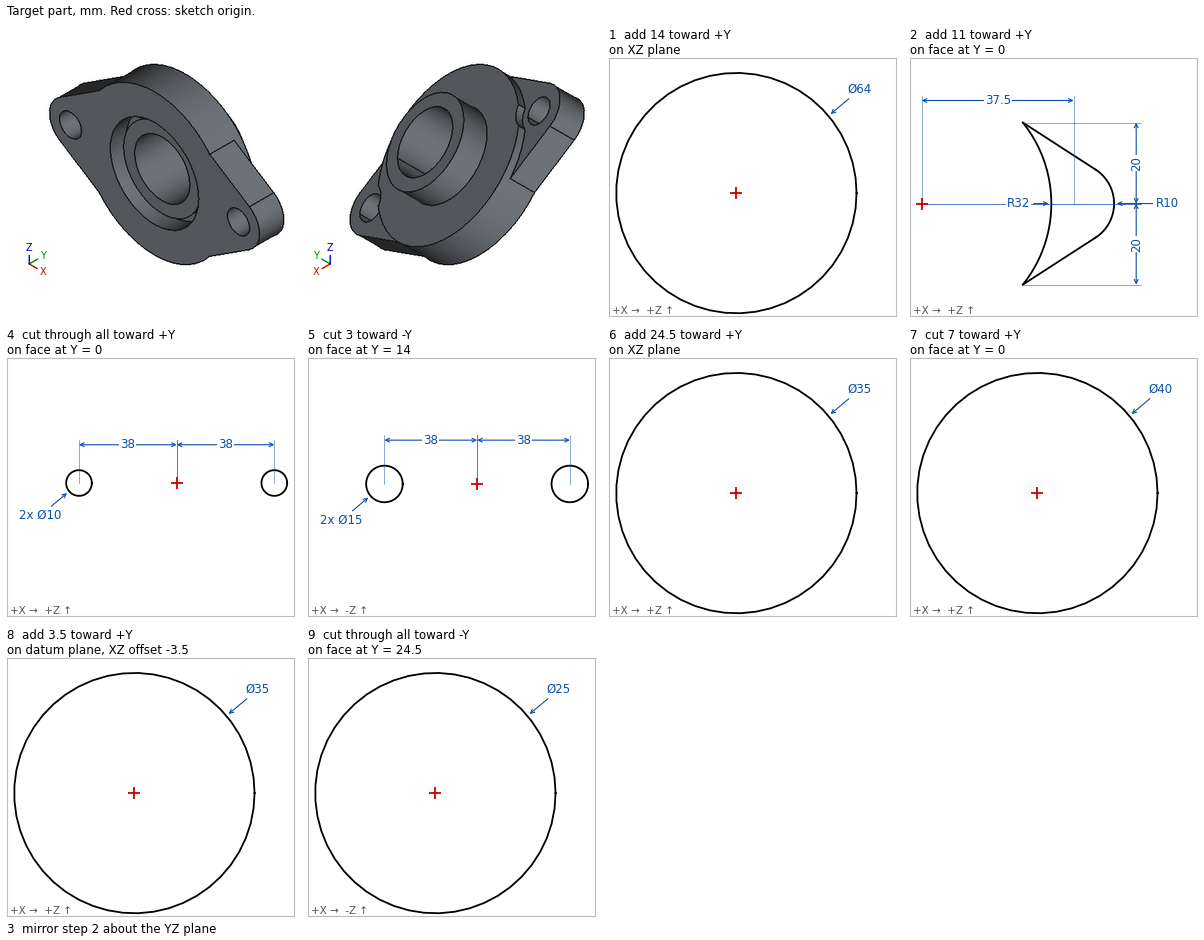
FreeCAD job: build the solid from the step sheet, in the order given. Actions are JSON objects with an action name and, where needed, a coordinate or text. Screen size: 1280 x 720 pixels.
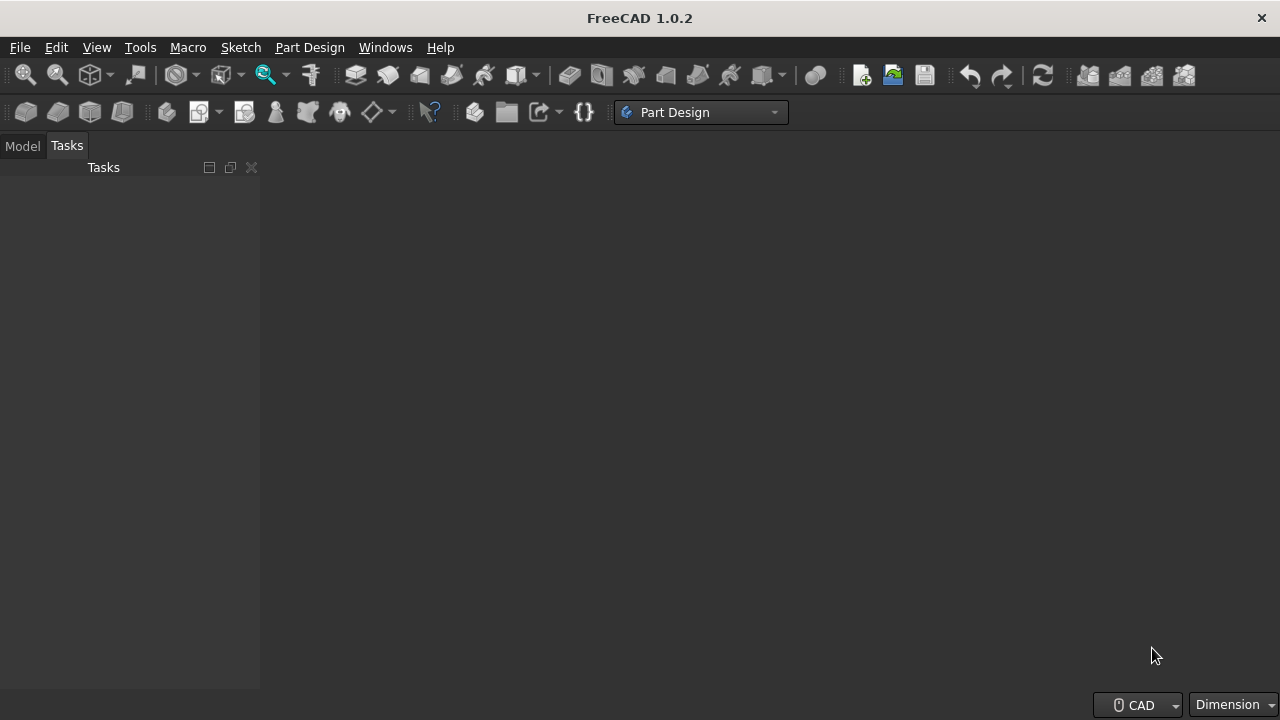
{"action": "left_click", "coordinate": [862, 76]}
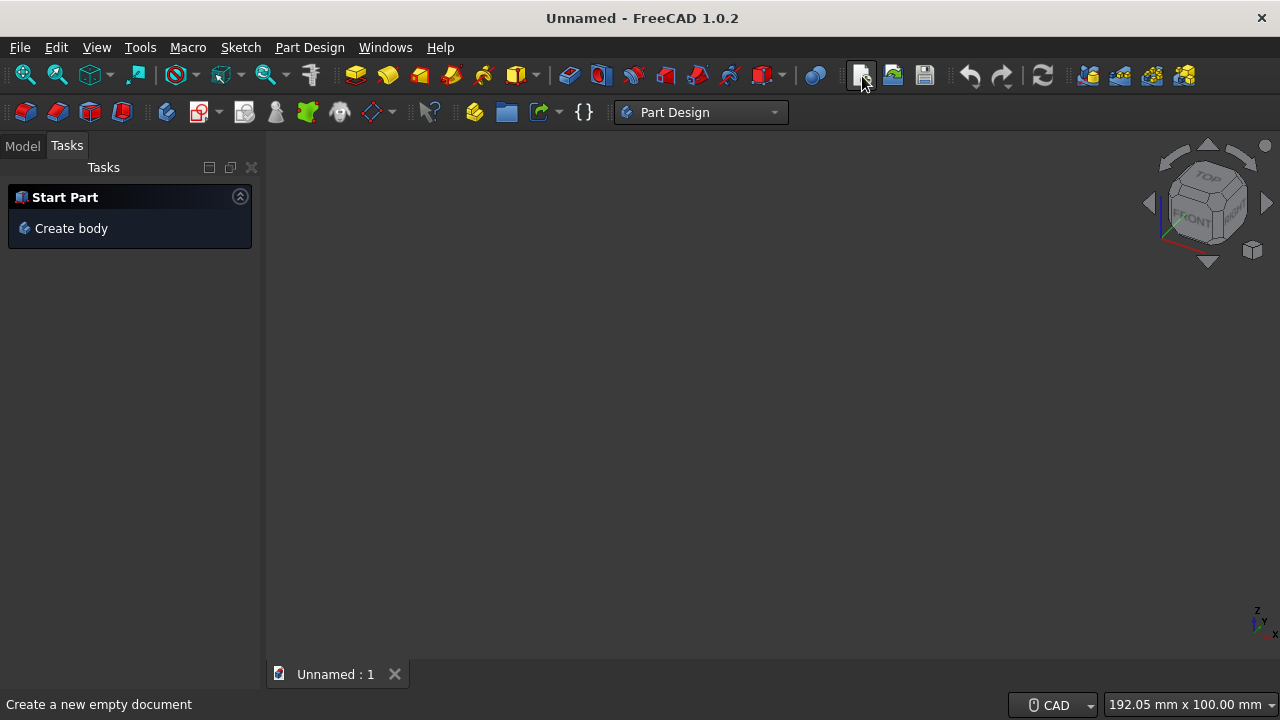
{"action": "left_click", "coordinate": [200, 112]}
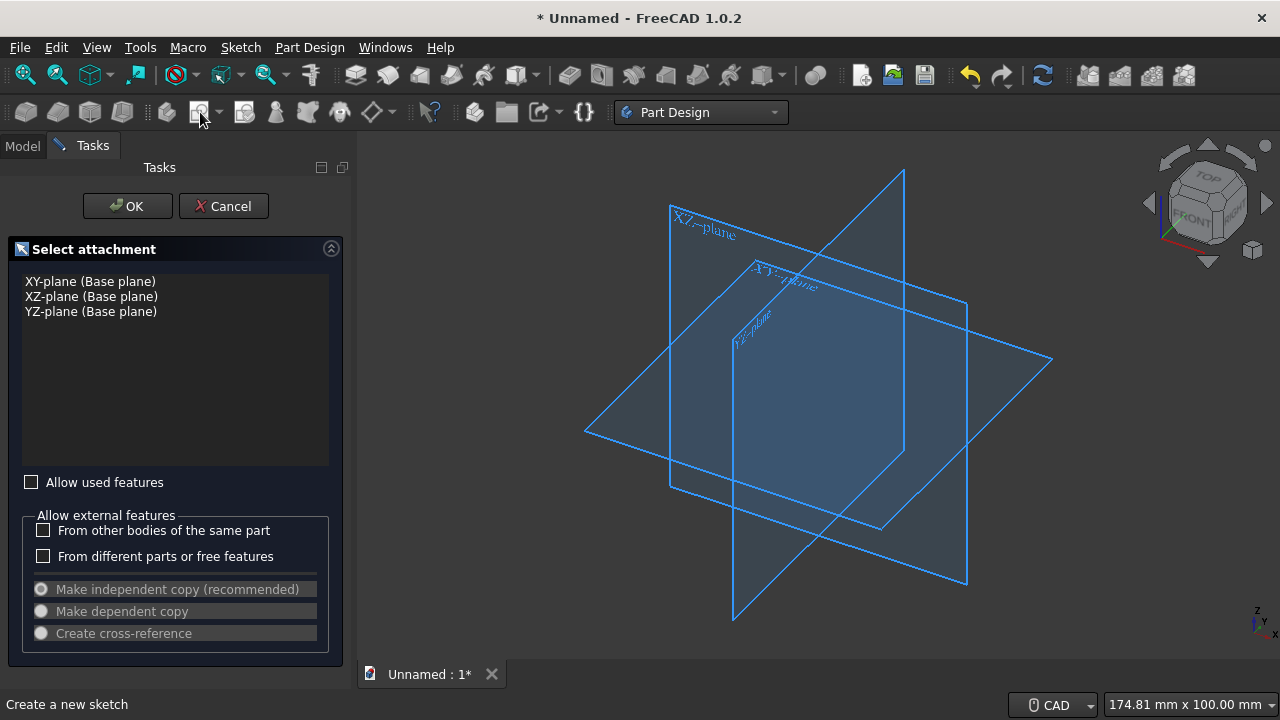
{"action": "left_click", "coordinate": [82, 296]}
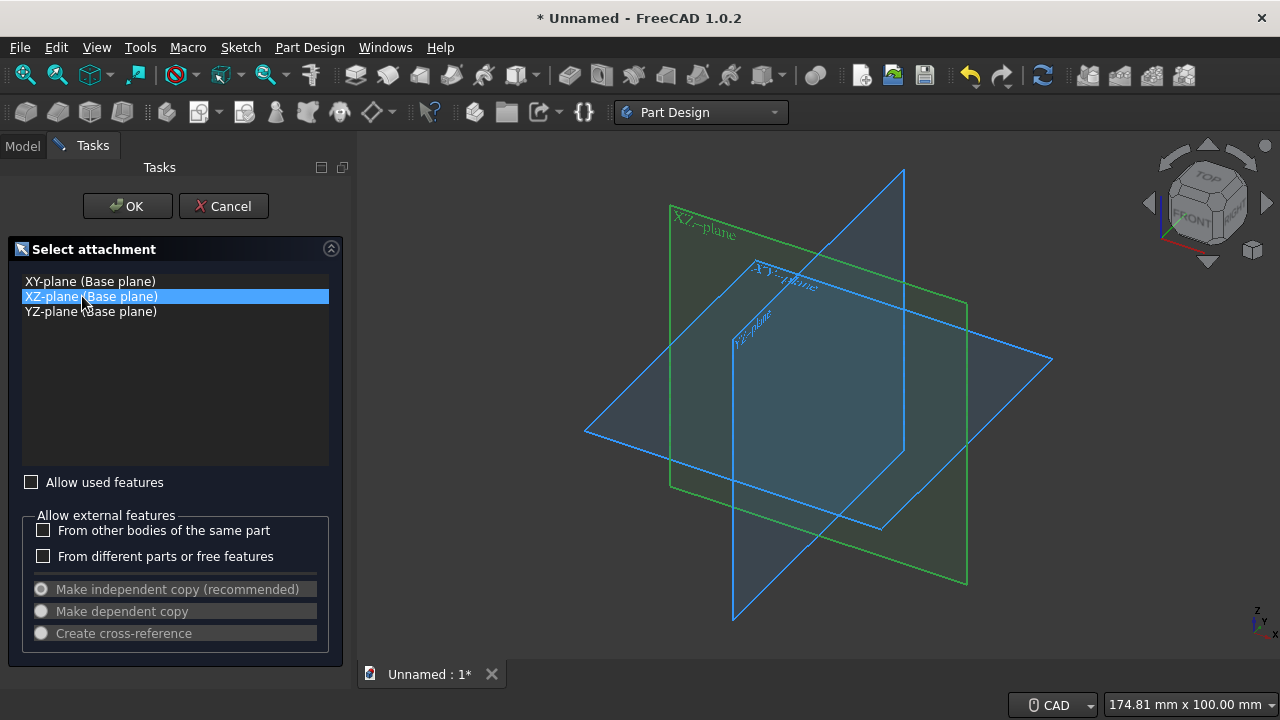
{"action": "left_click", "coordinate": [128, 206]}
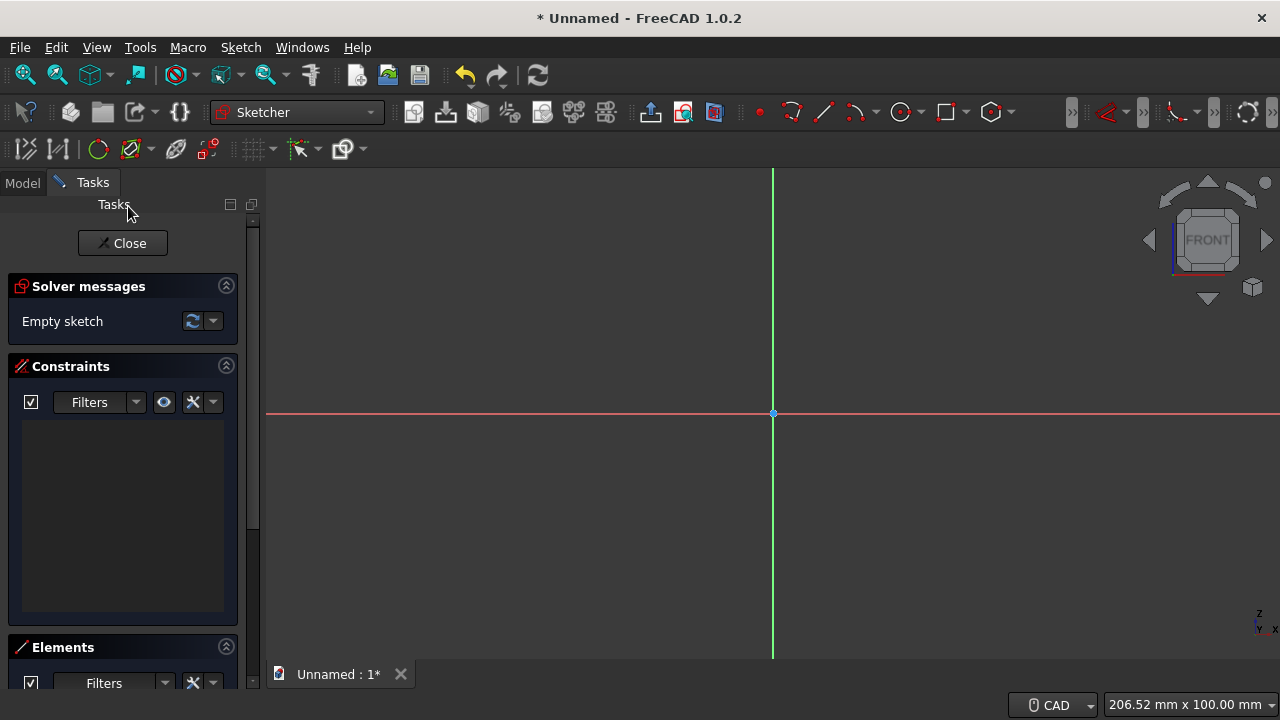
{"action": "key", "text": "g c"}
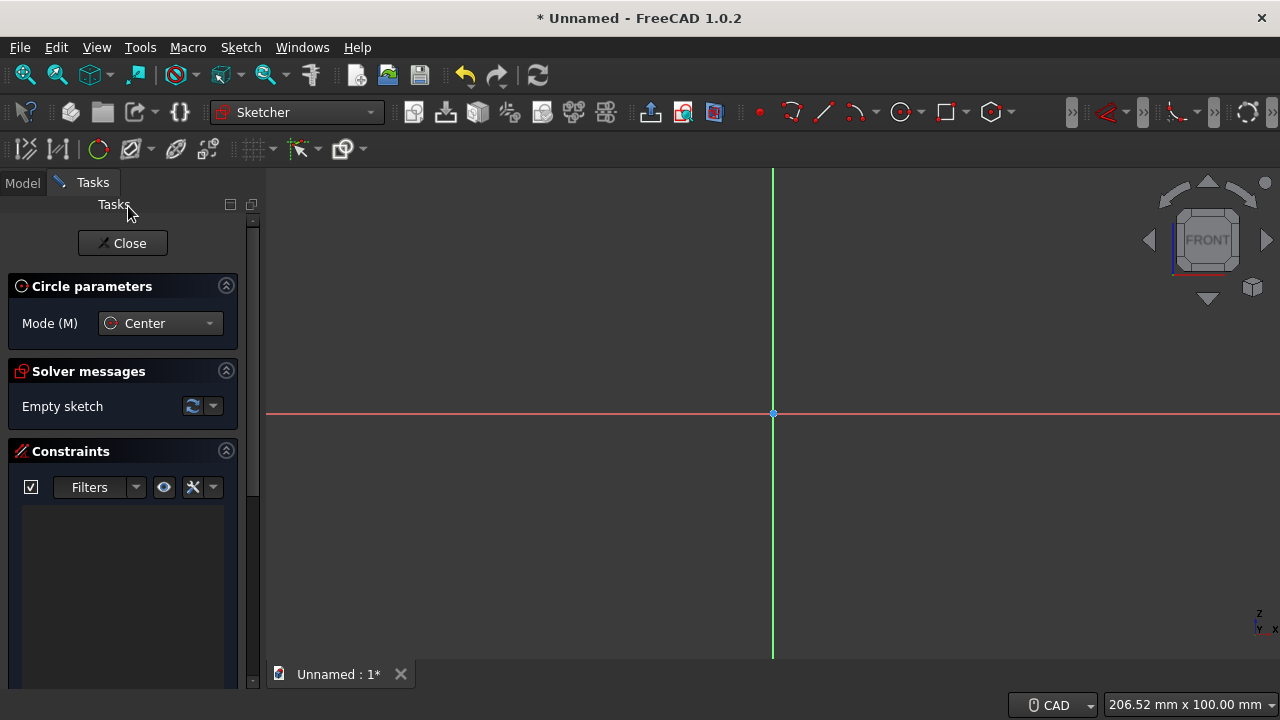
{"action": "left_click", "coordinate": [773, 414]}
{"action": "left_click", "coordinate": [884, 302]}
{"action": "key", "text": "Escape"}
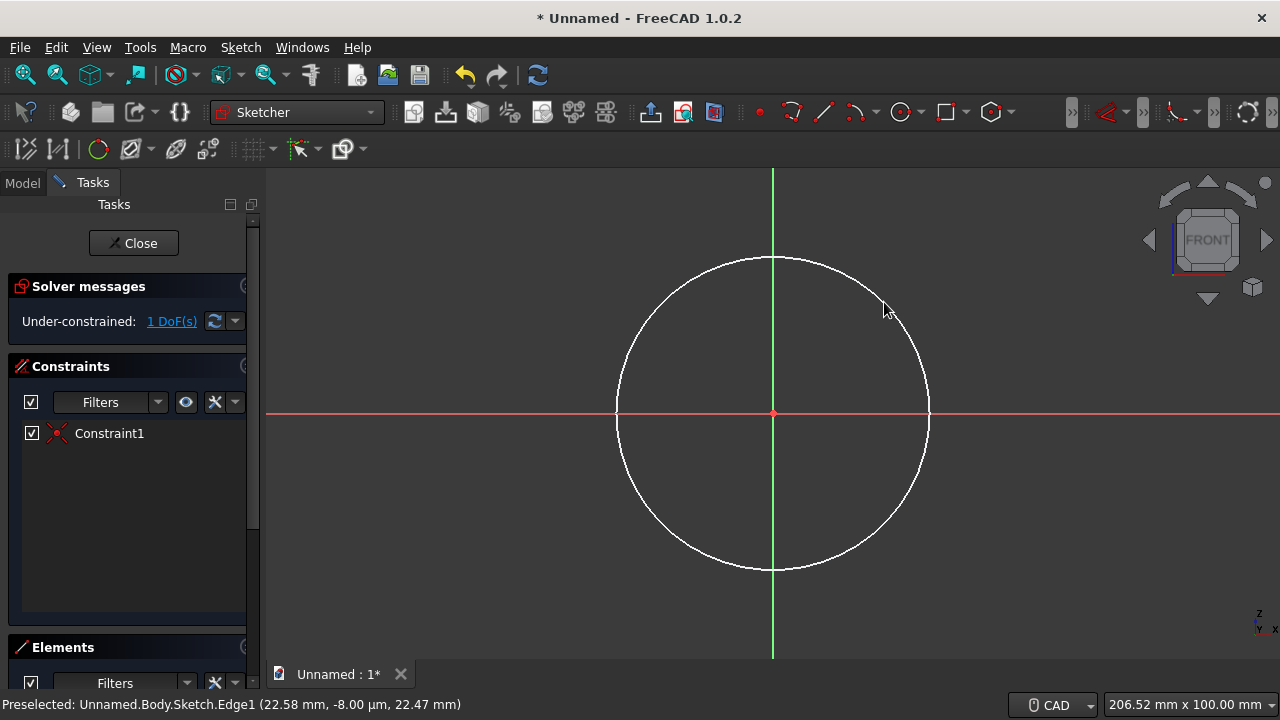
{"action": "left_click", "coordinate": [1106, 112]}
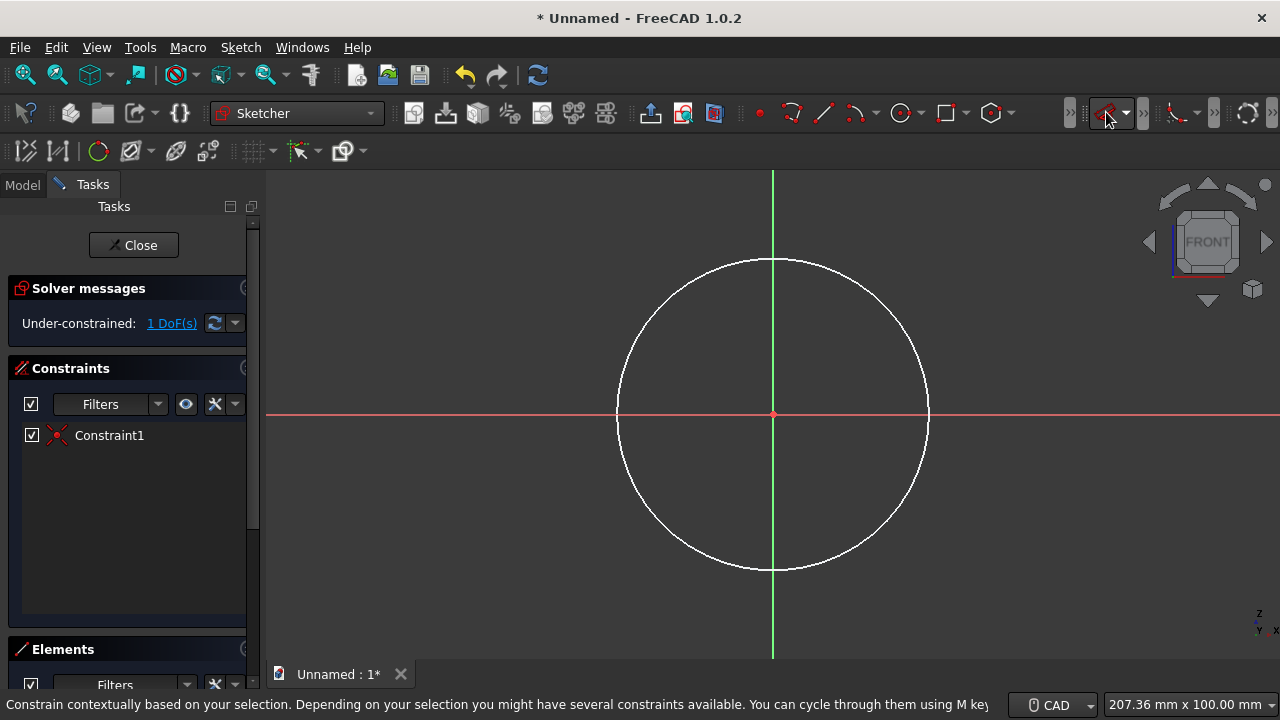
{"action": "left_click", "coordinate": [883, 304]}
{"action": "left_click", "coordinate": [906, 281]}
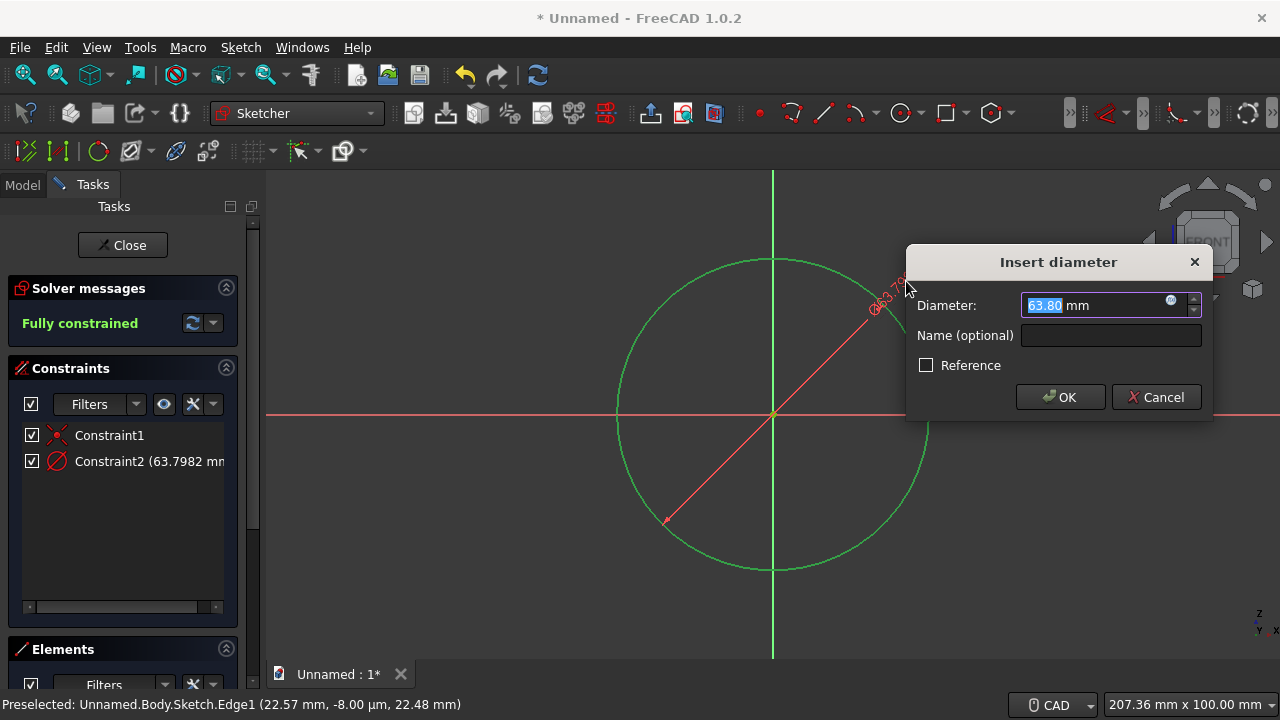
{"action": "type", "text": "64"}
{"action": "key", "text": "Return"}
{"action": "key", "text": "Escape"}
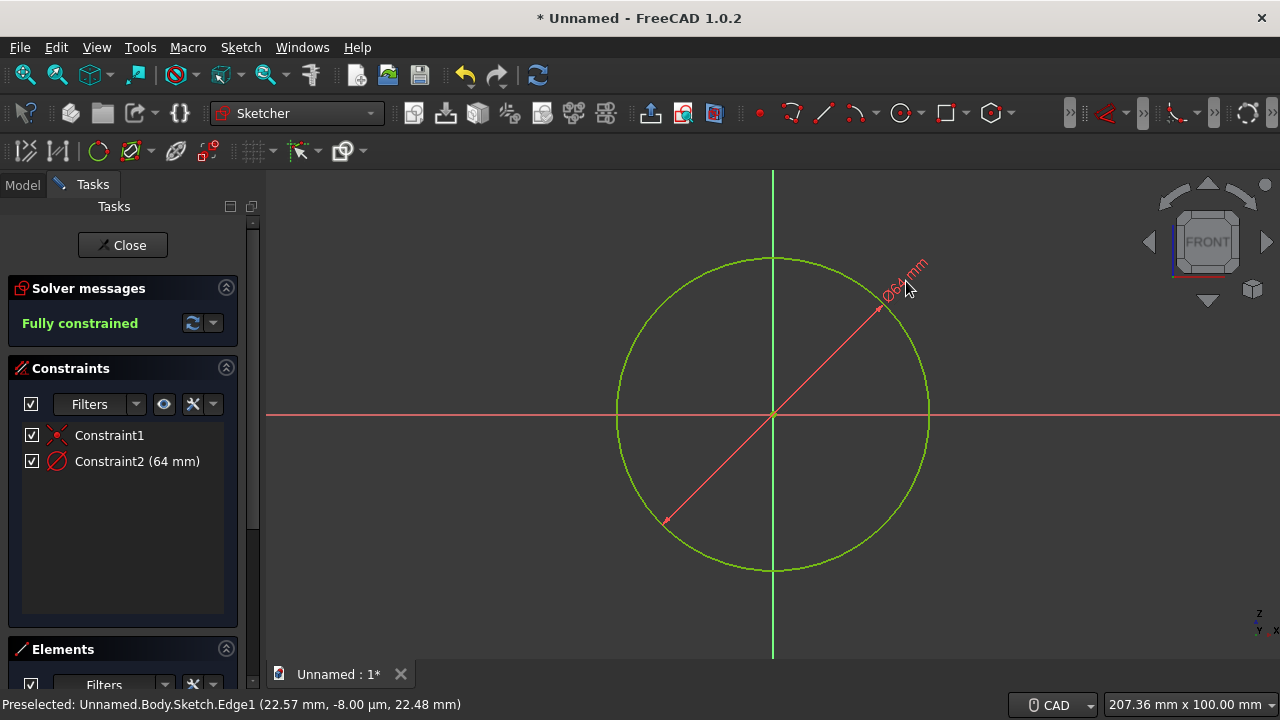
{"action": "left_click", "coordinate": [123, 245]}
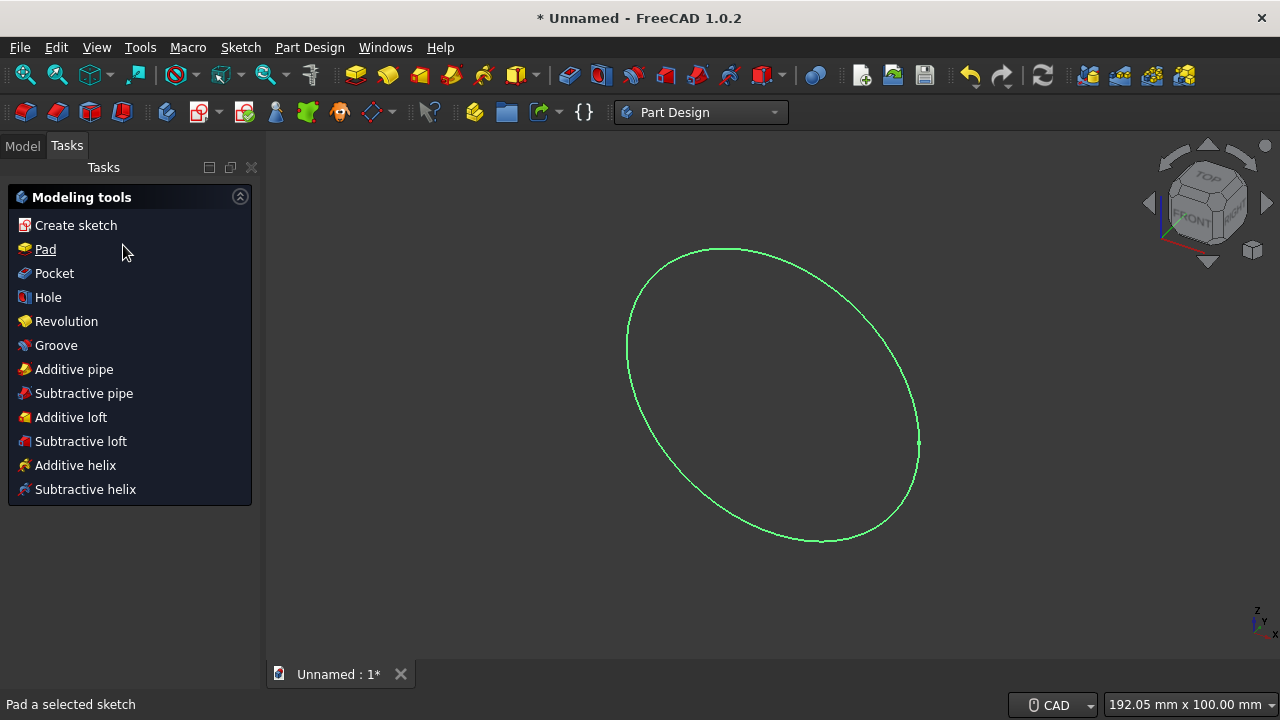
{"action": "left_click", "coordinate": [356, 76]}